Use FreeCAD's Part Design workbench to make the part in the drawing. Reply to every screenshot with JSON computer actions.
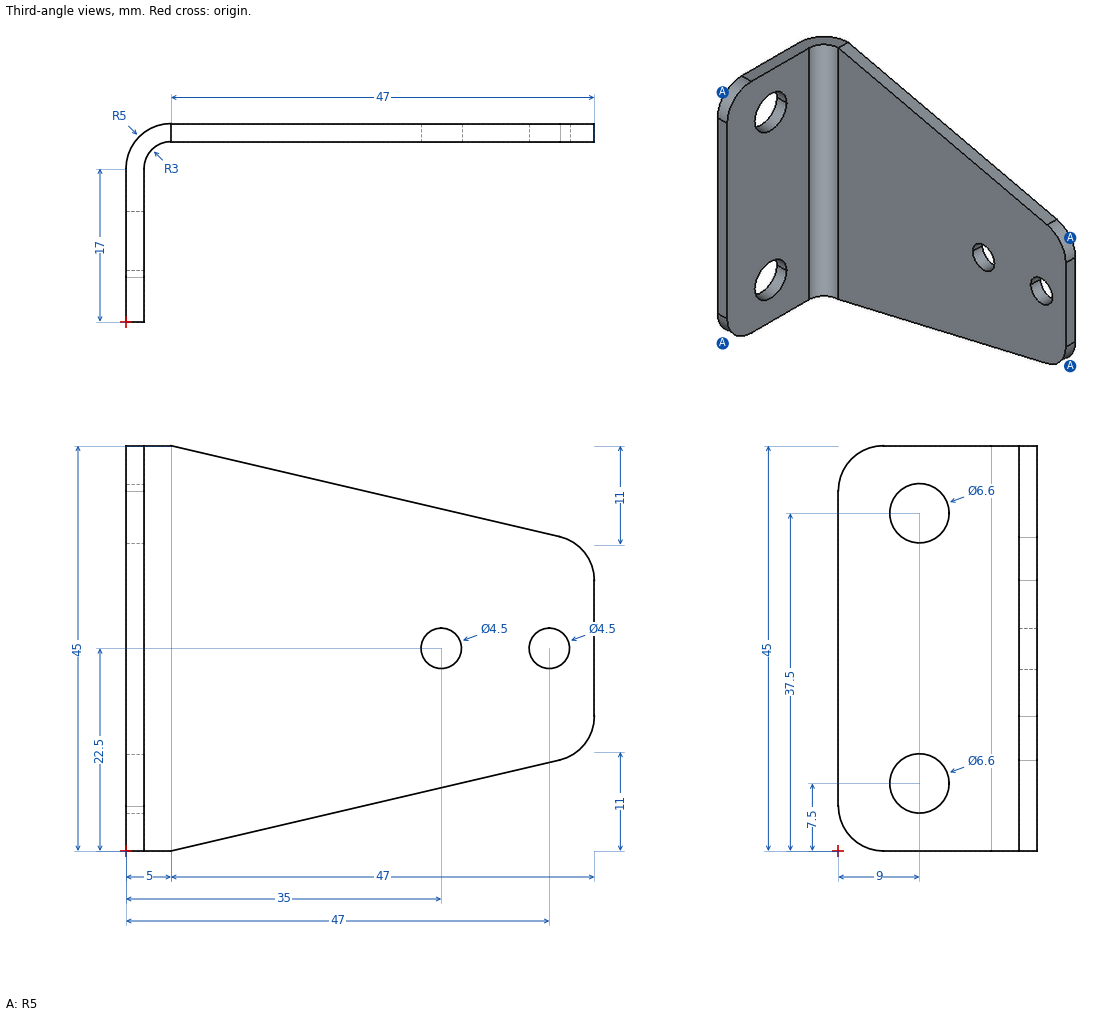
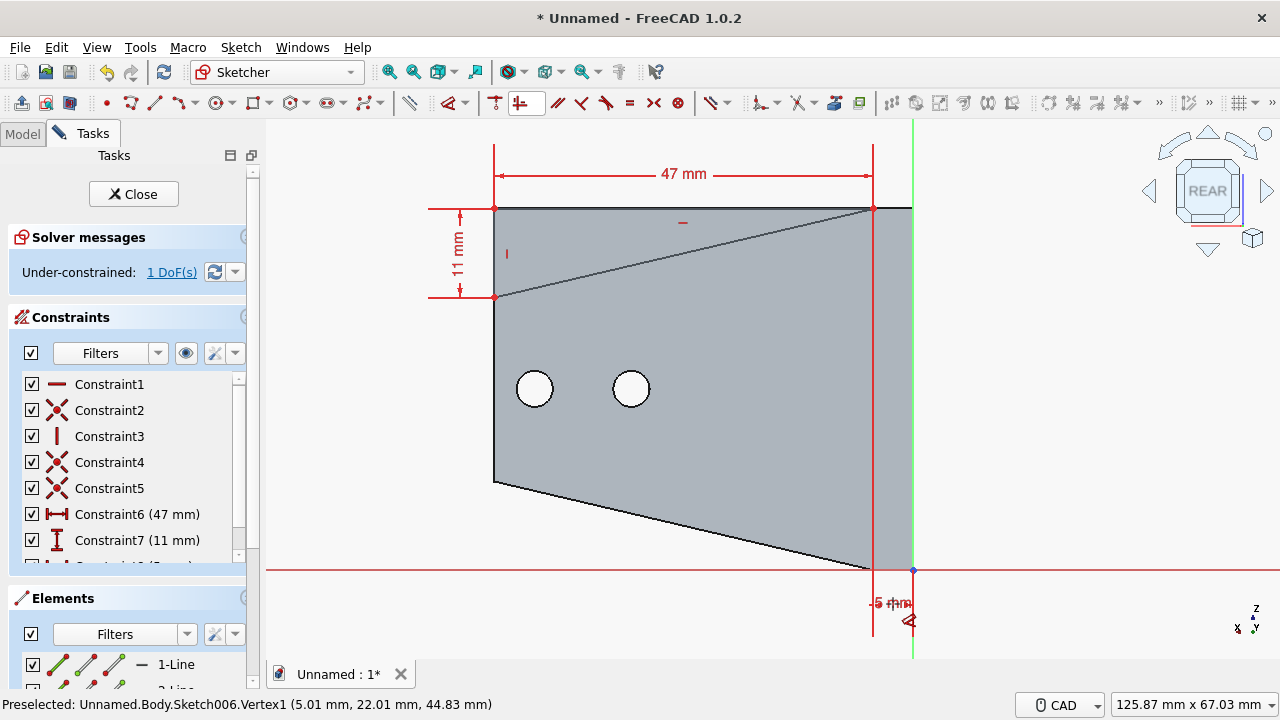
{"action": "left_click", "coordinate": [873, 209]}
{"action": "left_click", "coordinate": [947, 390]}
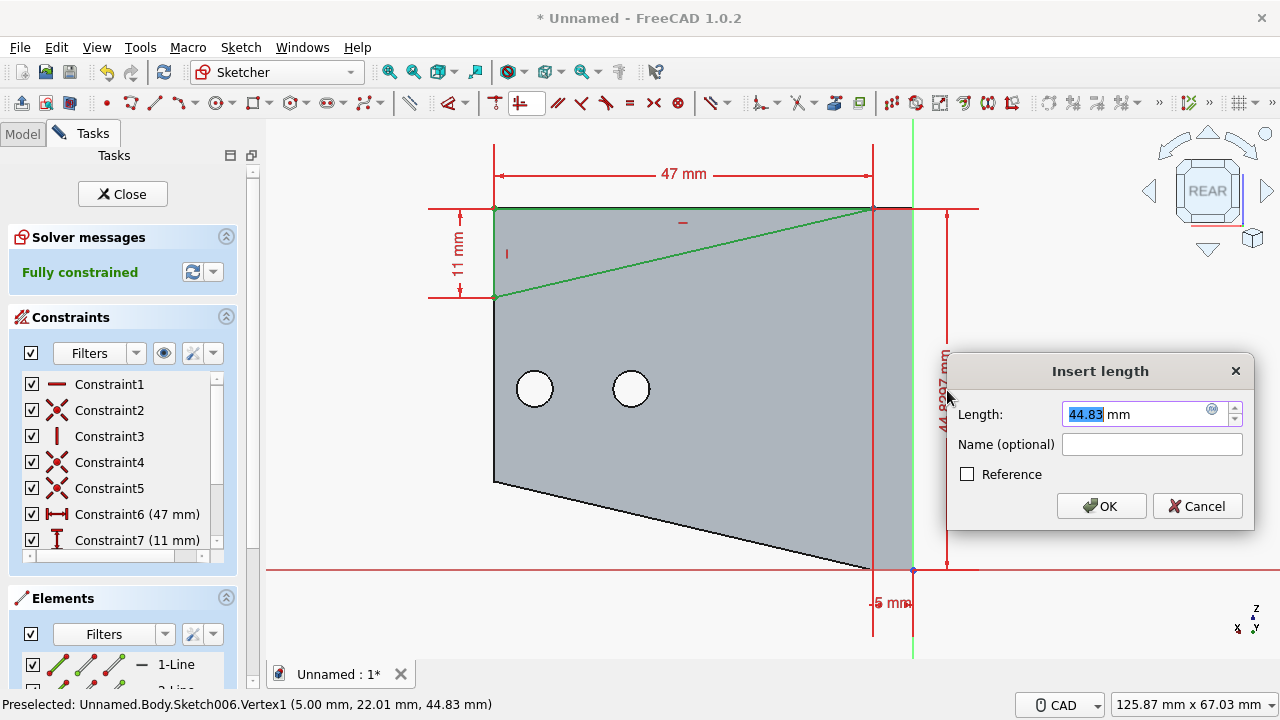
{"action": "type", "text": "45"}
{"action": "key", "text": "Return"}
{"action": "key", "text": "Escape"}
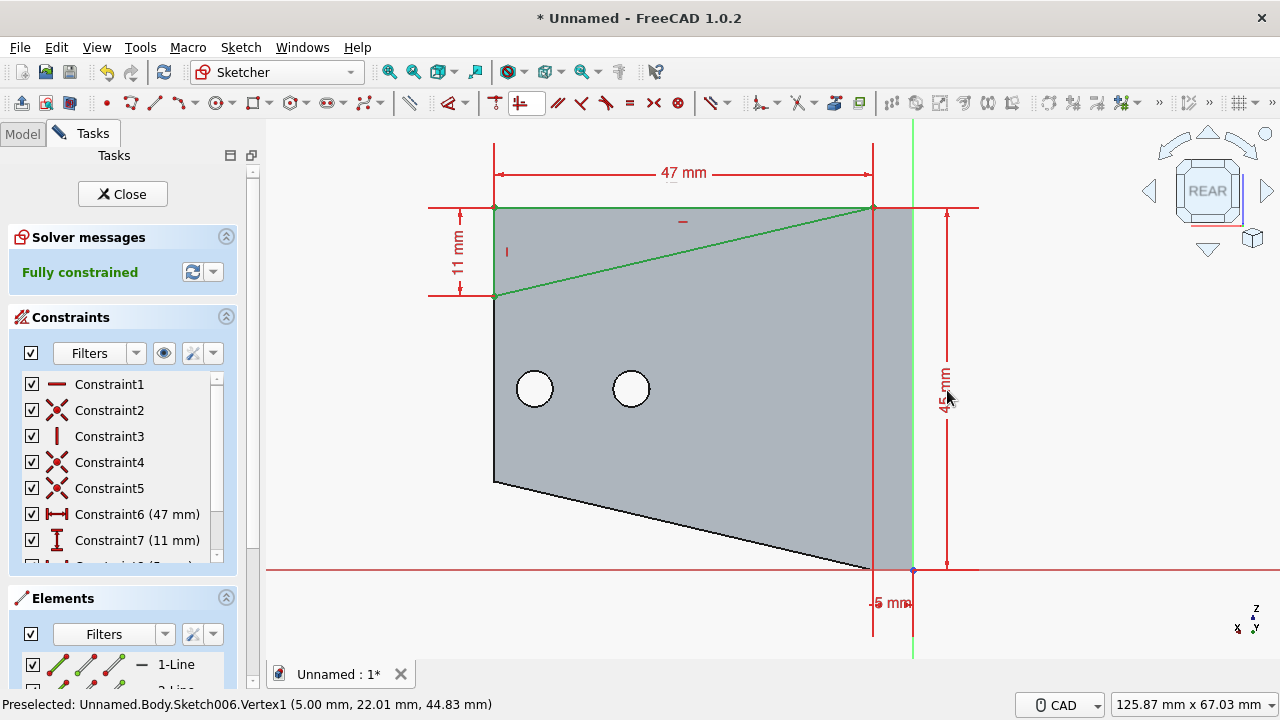
{"action": "left_click", "coordinate": [123, 194]}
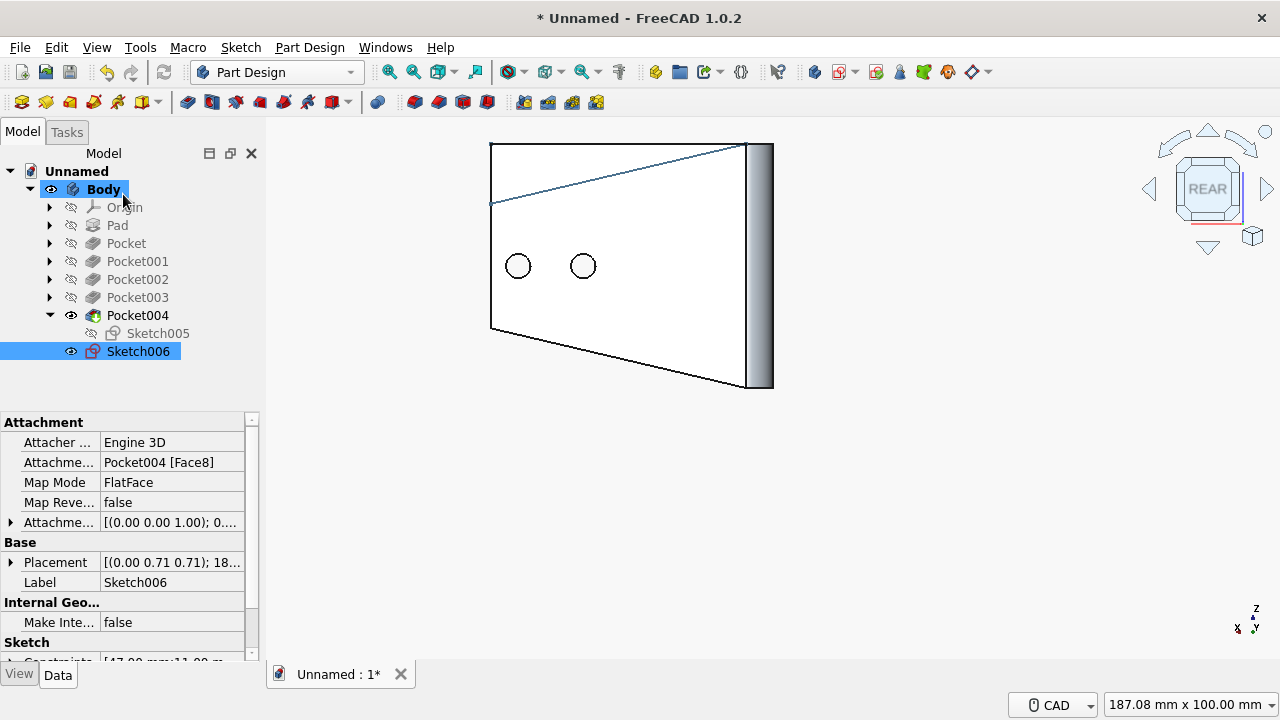
{"action": "left_click", "coordinate": [188, 102]}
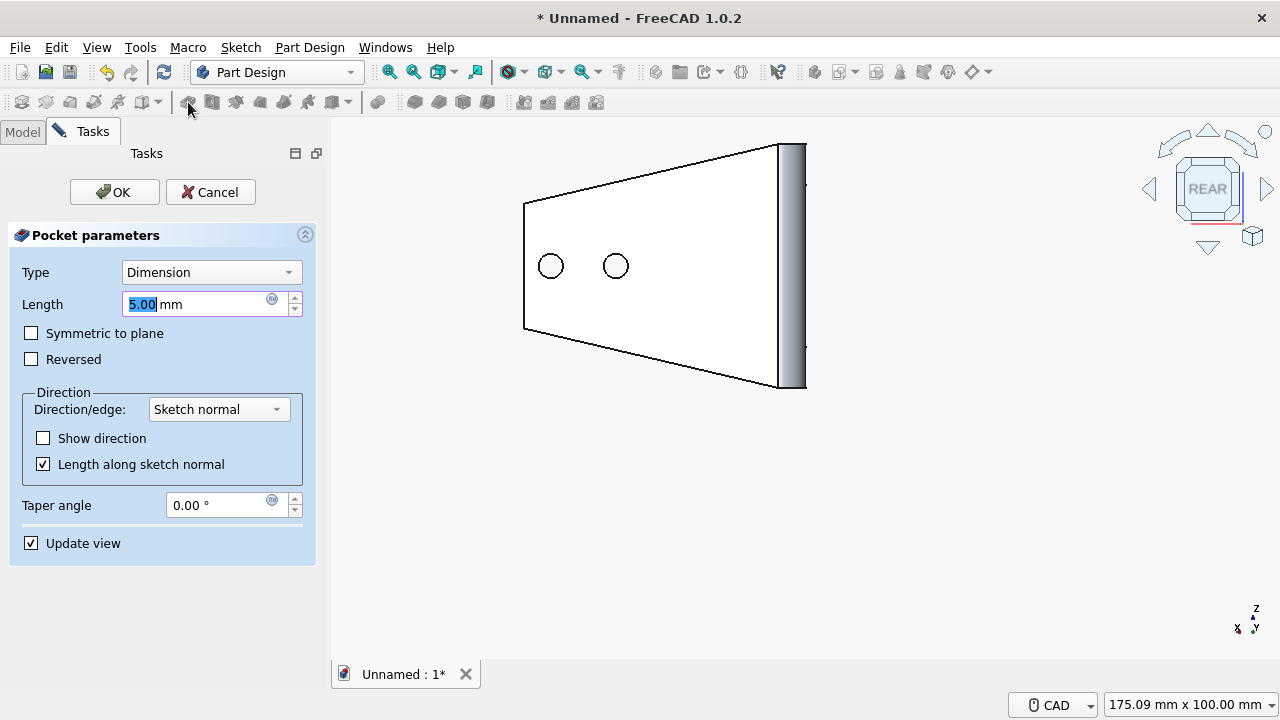
{"action": "left_click", "coordinate": [212, 272]}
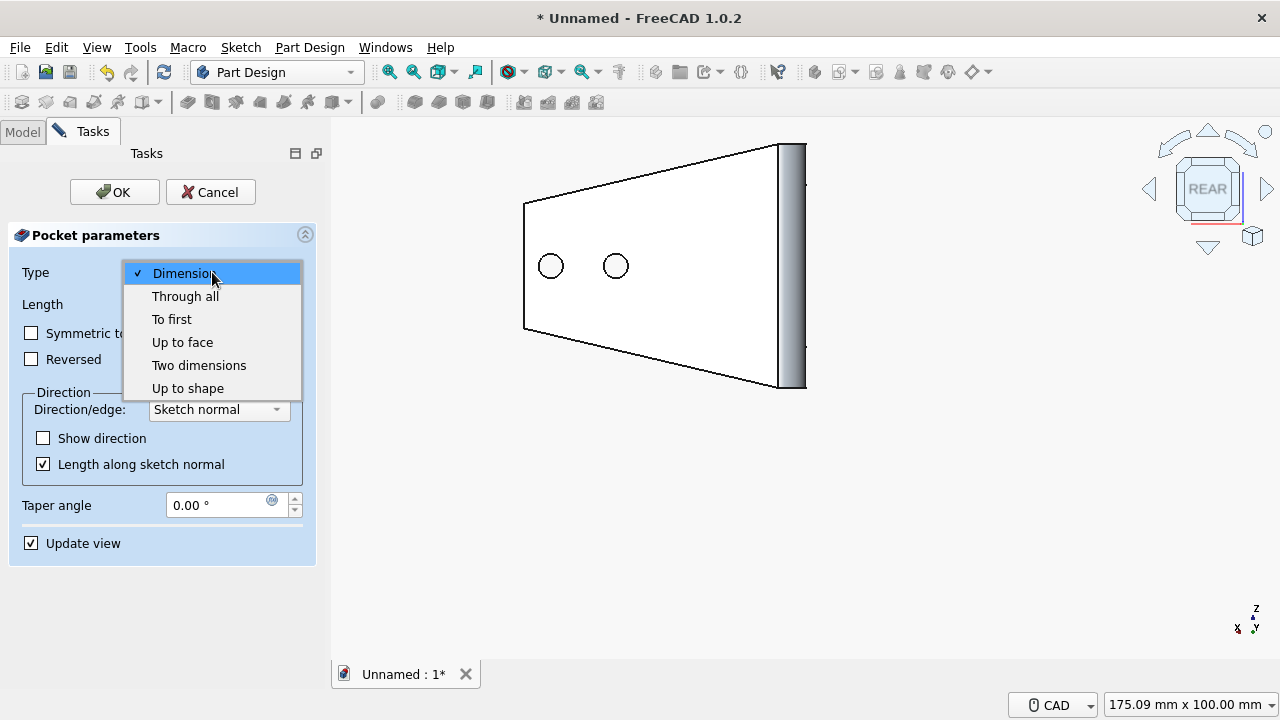
{"action": "left_click", "coordinate": [212, 320]}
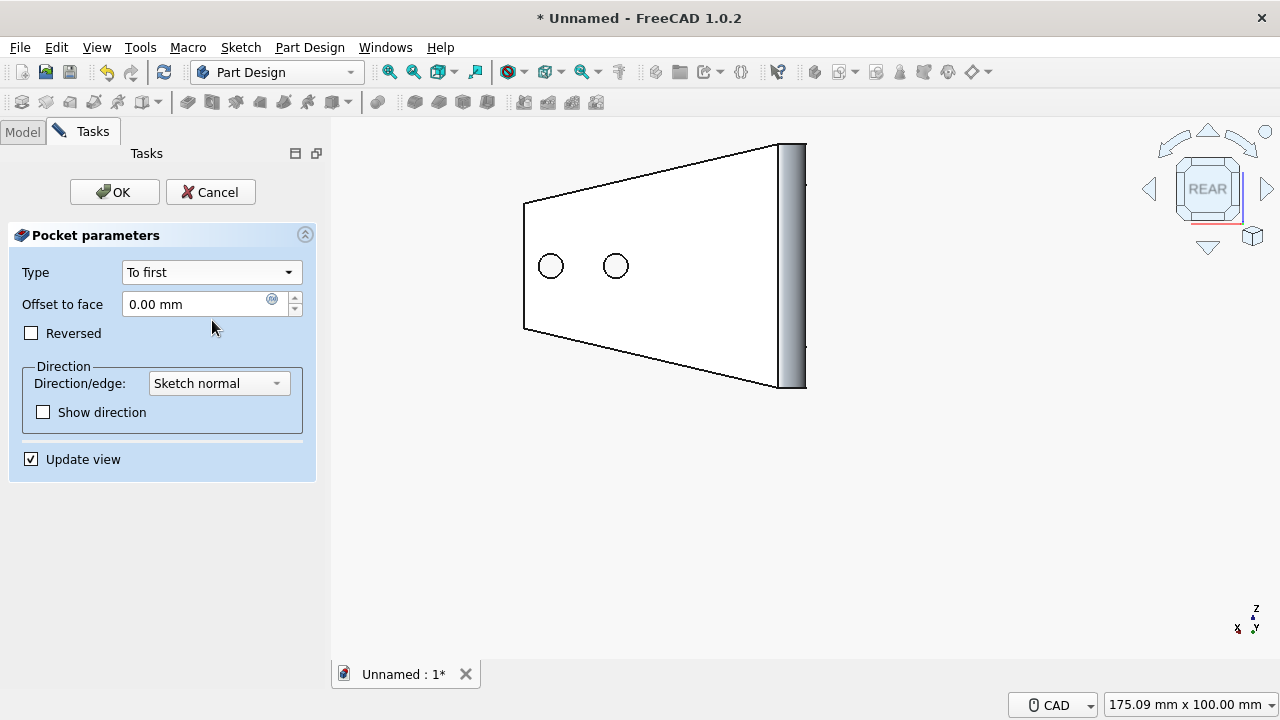
{"action": "left_click", "coordinate": [115, 192]}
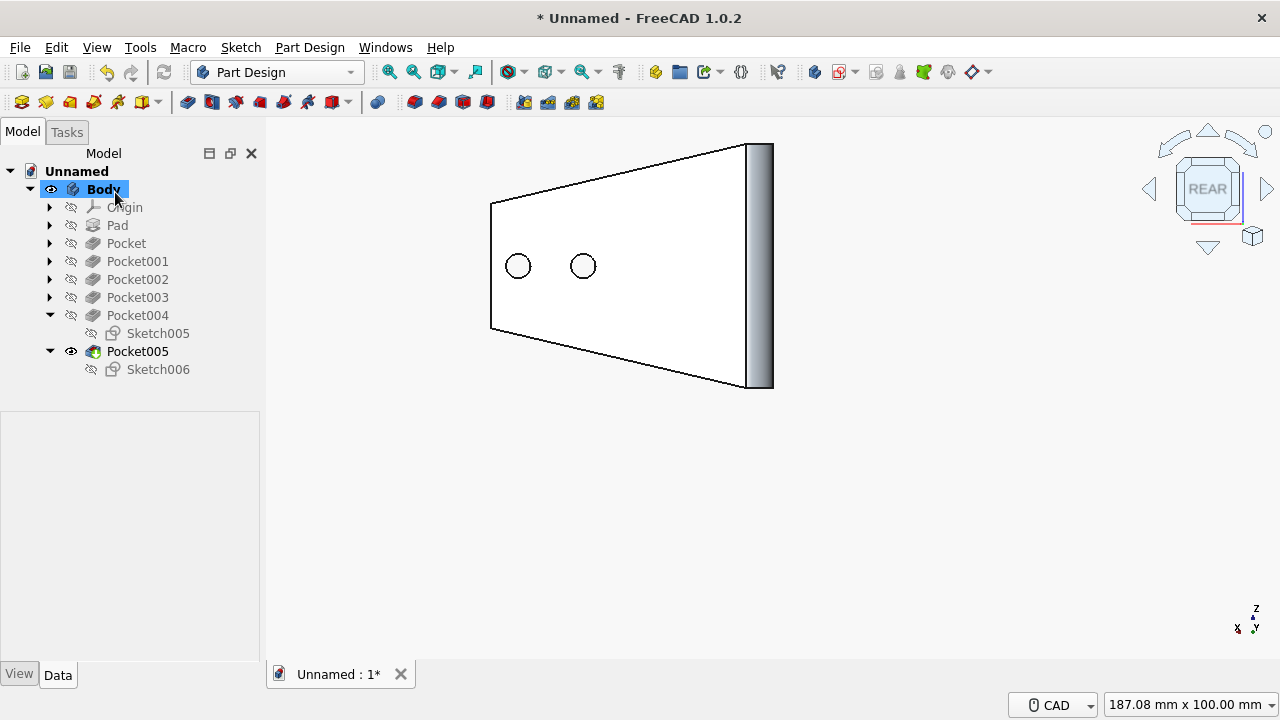
{"action": "scroll", "coordinate": [768, 387], "scroll_direction": "up", "scroll_amount": 7}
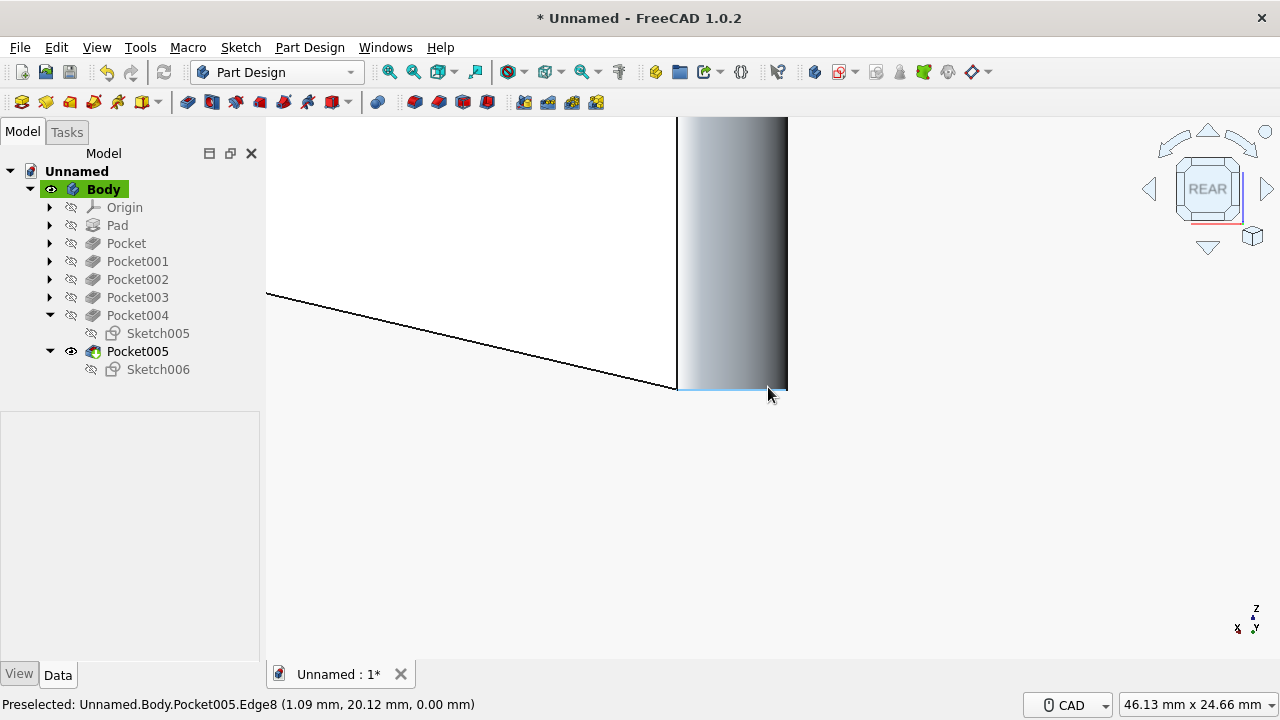
{"action": "key", "text": "v f"}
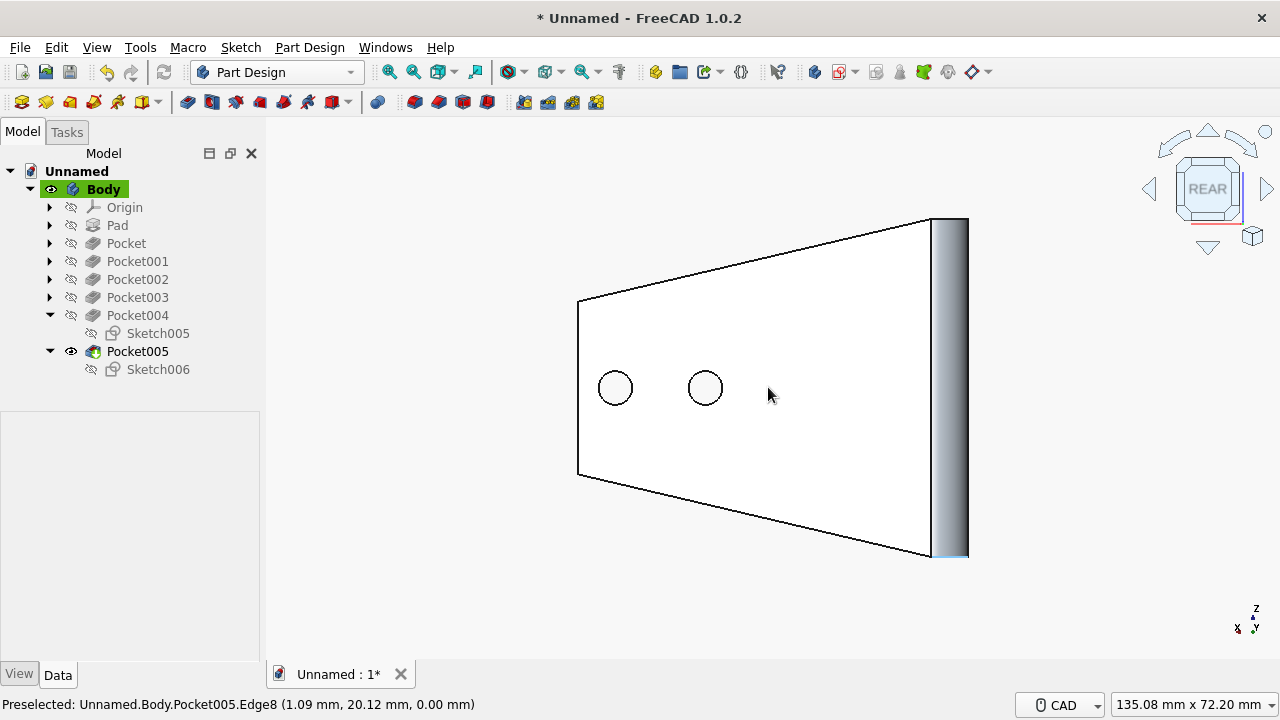
{"action": "key", "text": "0"}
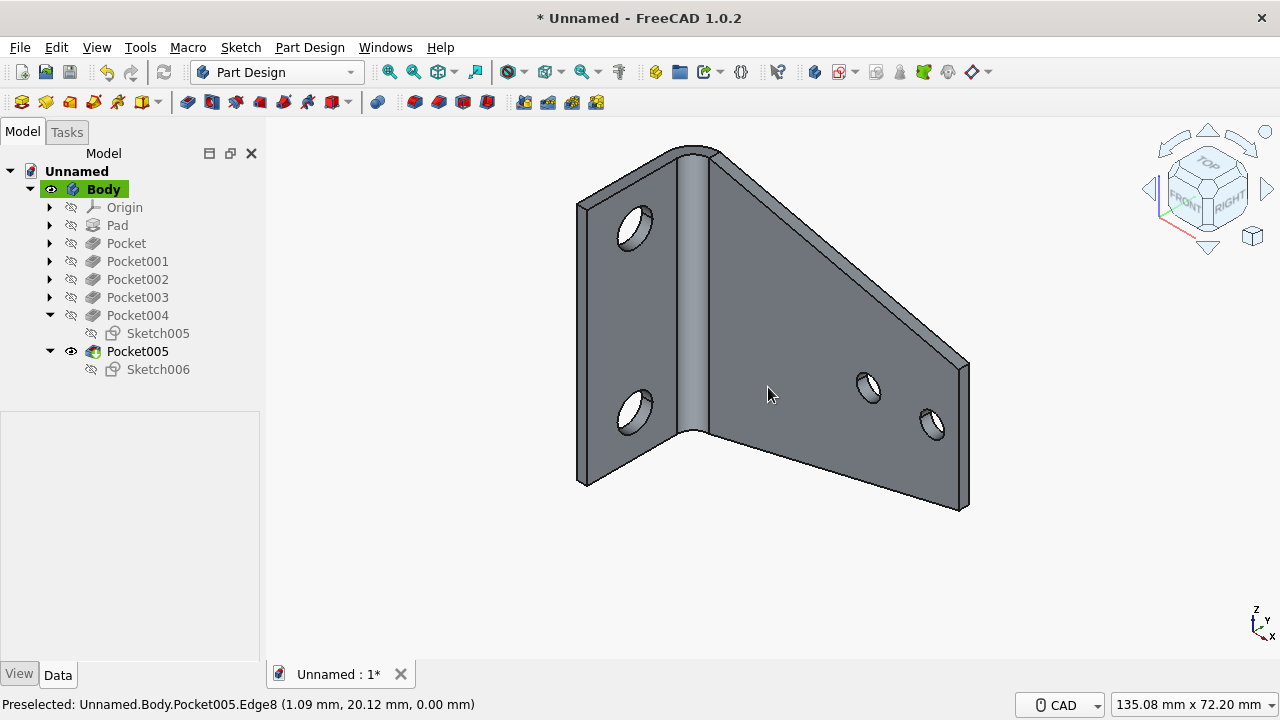
{"action": "left_click", "coordinate": [581, 206]}